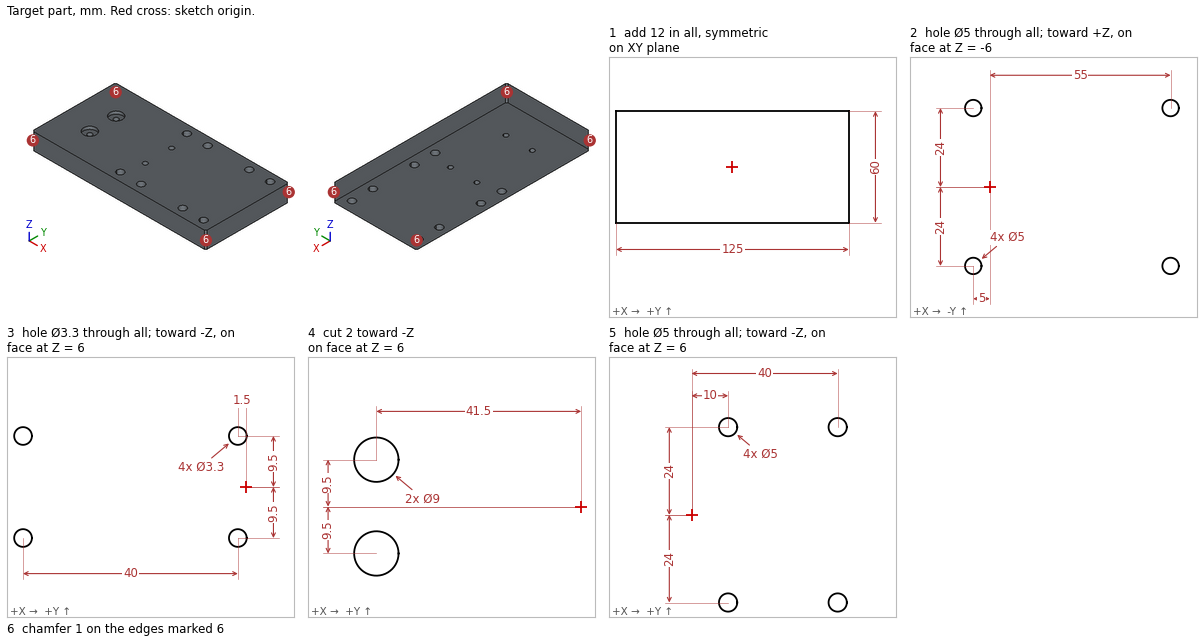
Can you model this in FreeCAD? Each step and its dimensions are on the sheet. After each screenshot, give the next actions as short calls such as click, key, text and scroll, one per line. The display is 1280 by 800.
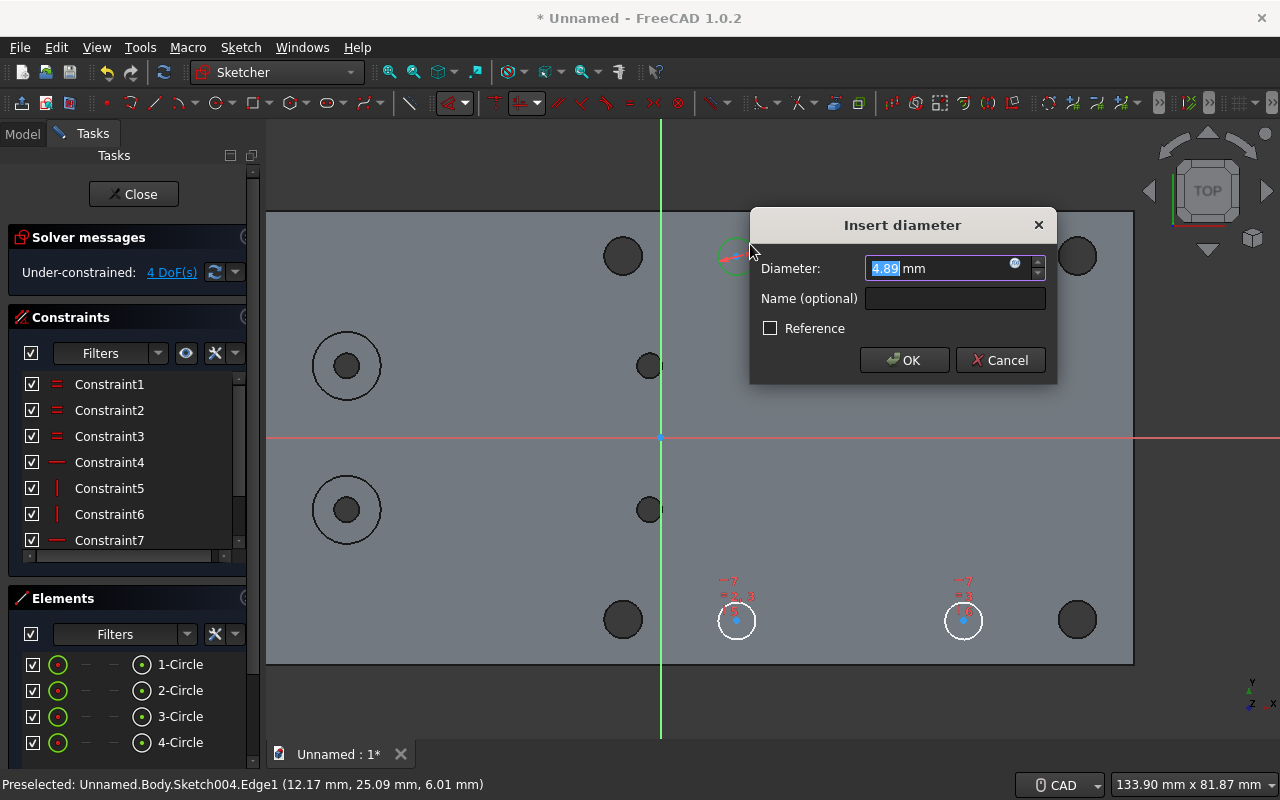
text(5)
key(Return)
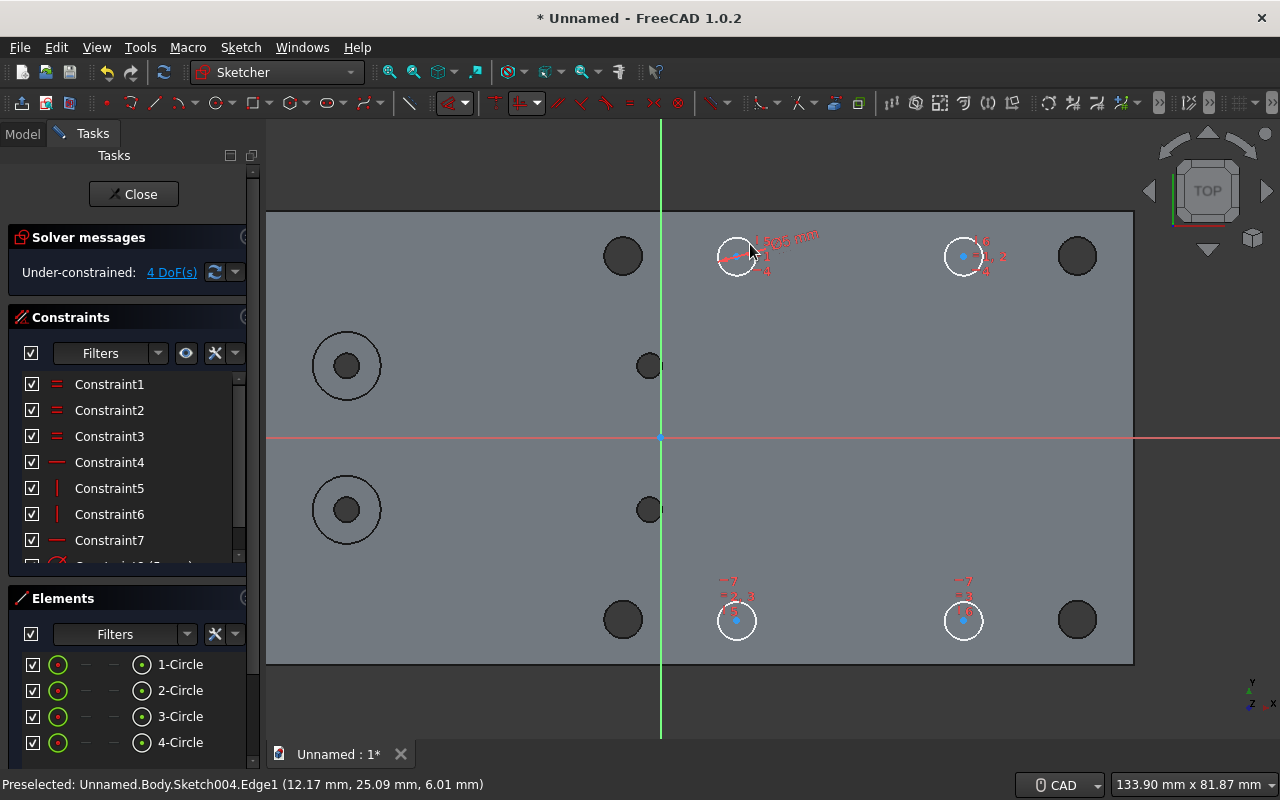
click(737, 257)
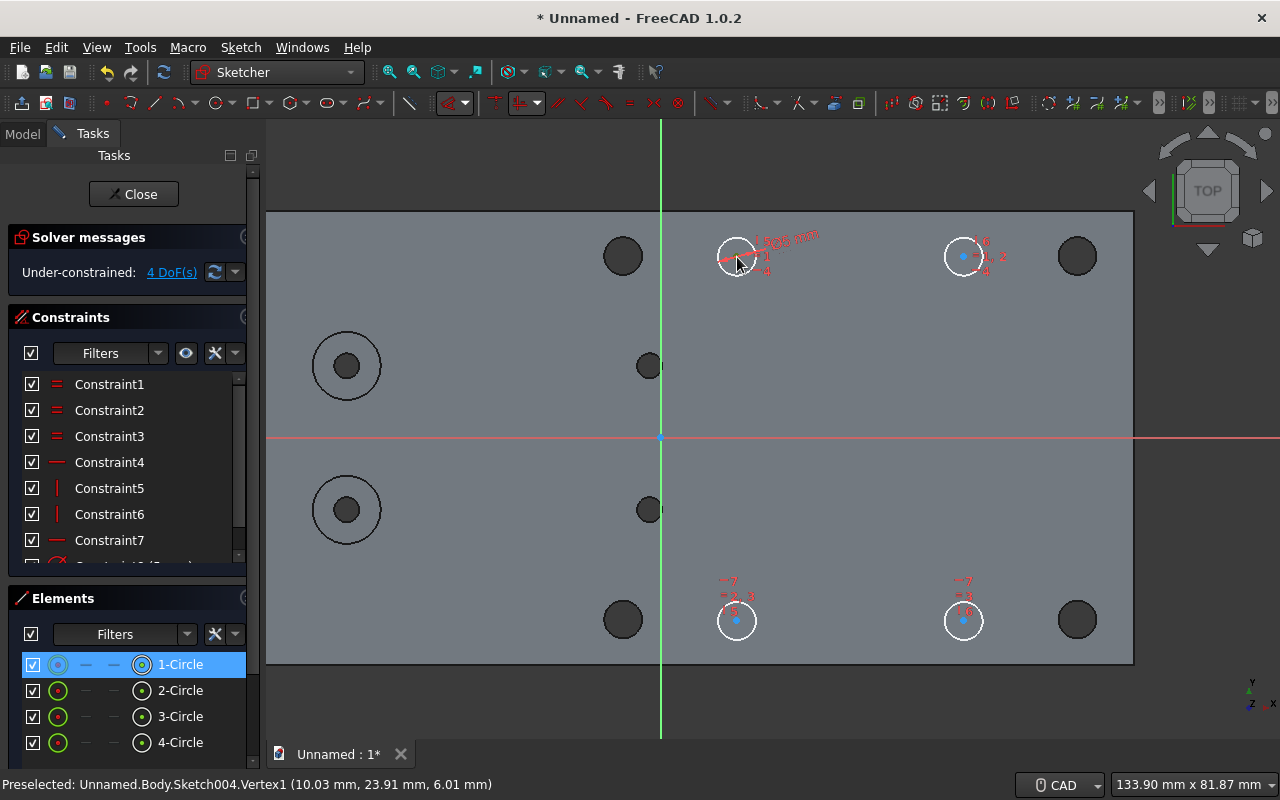
key(l)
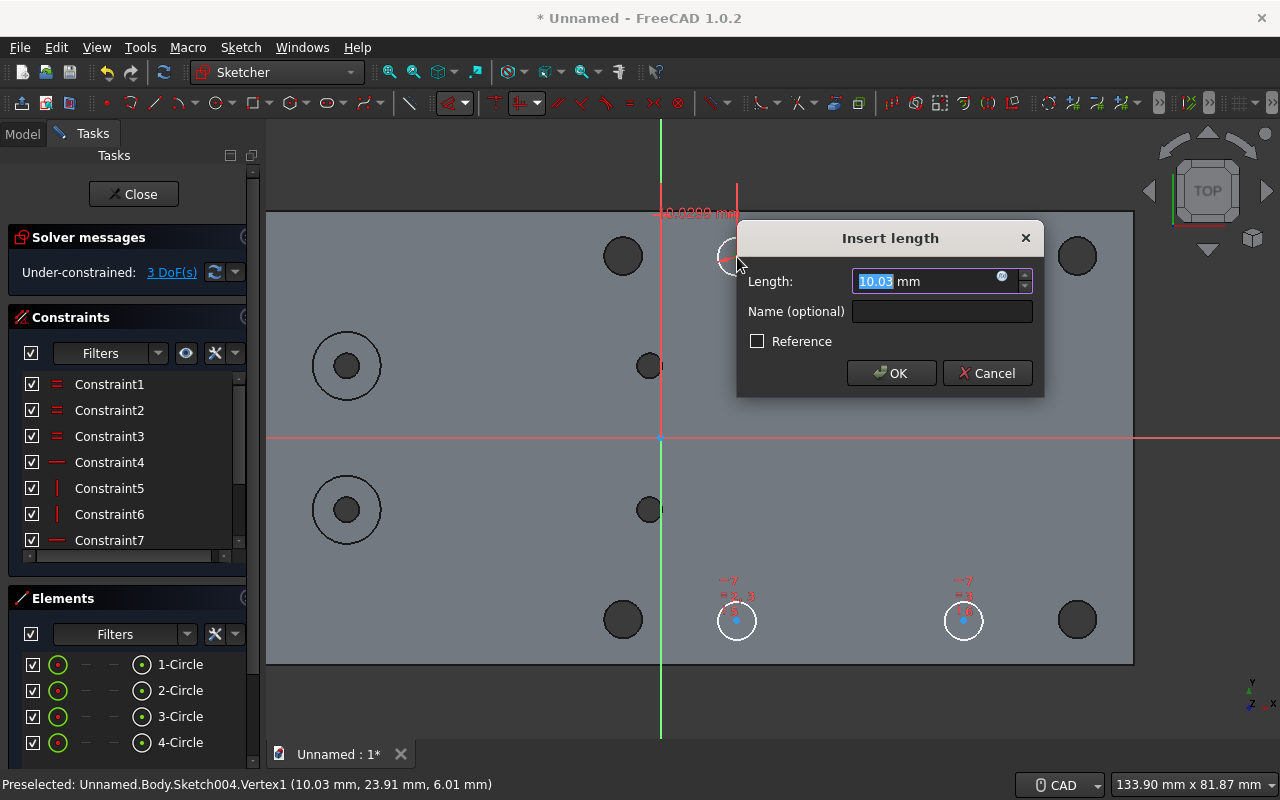
text(10)
key(Return)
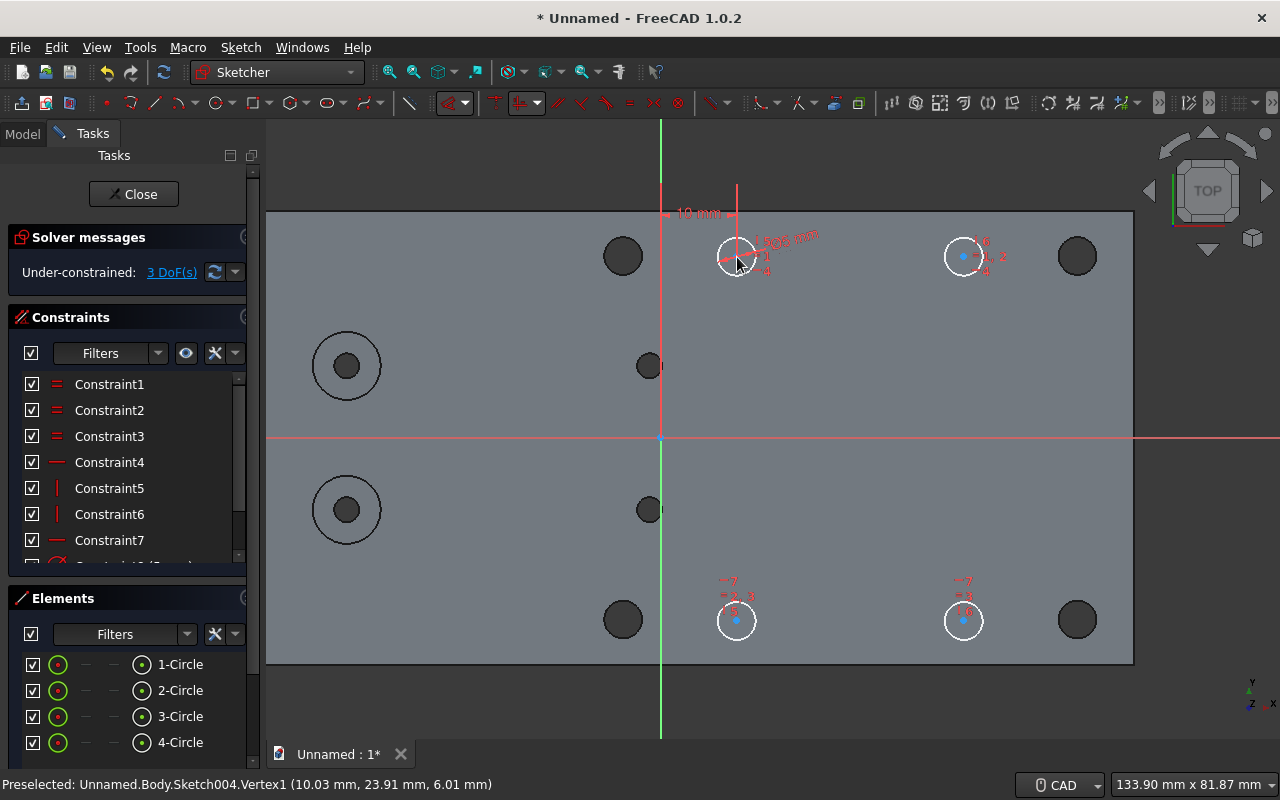
click(737, 257)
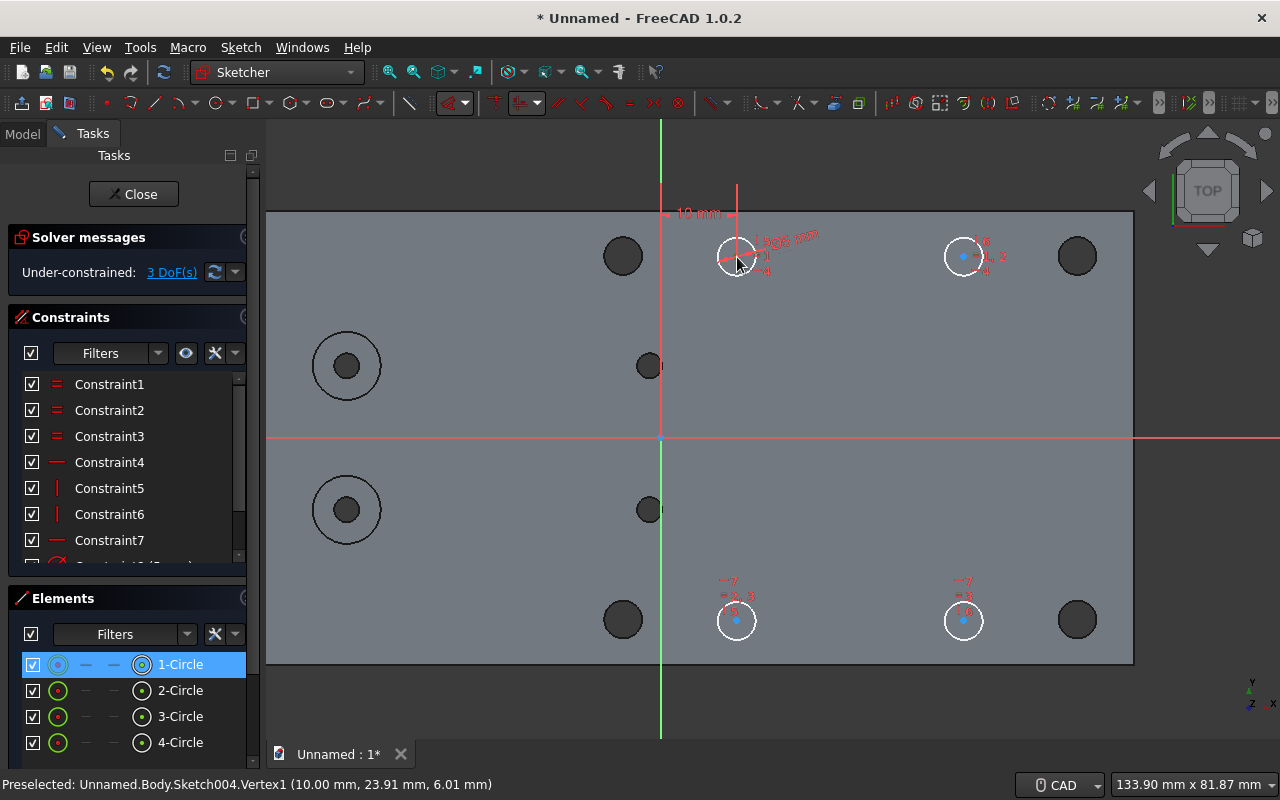
click(468, 104)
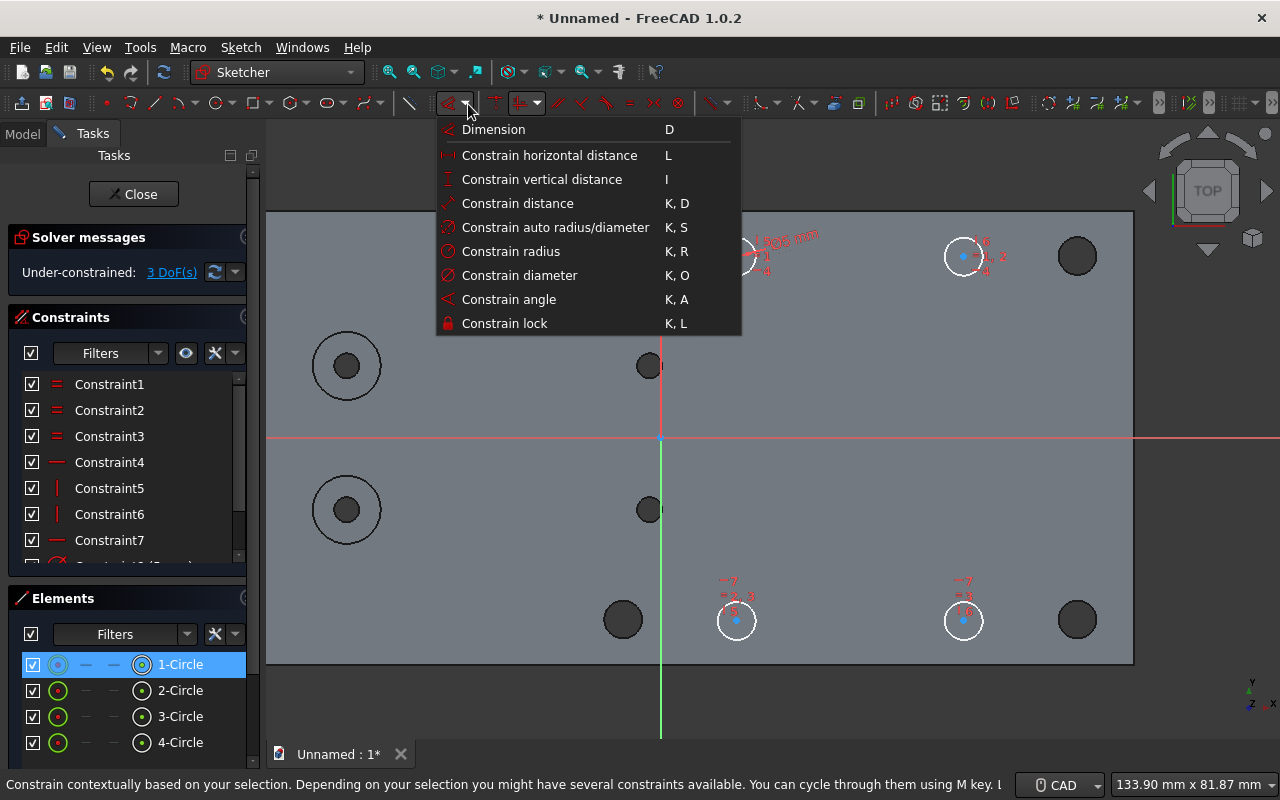
click(589, 179)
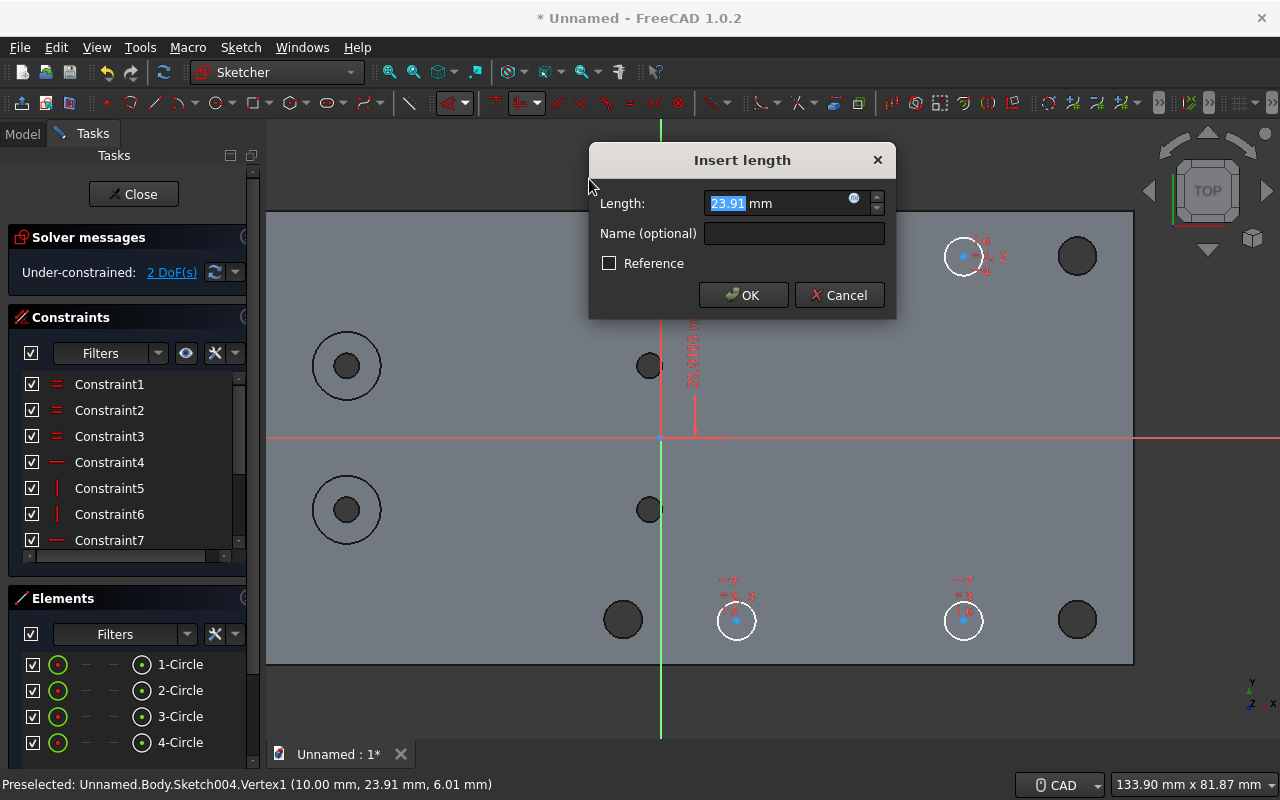
text(24)
key(Return)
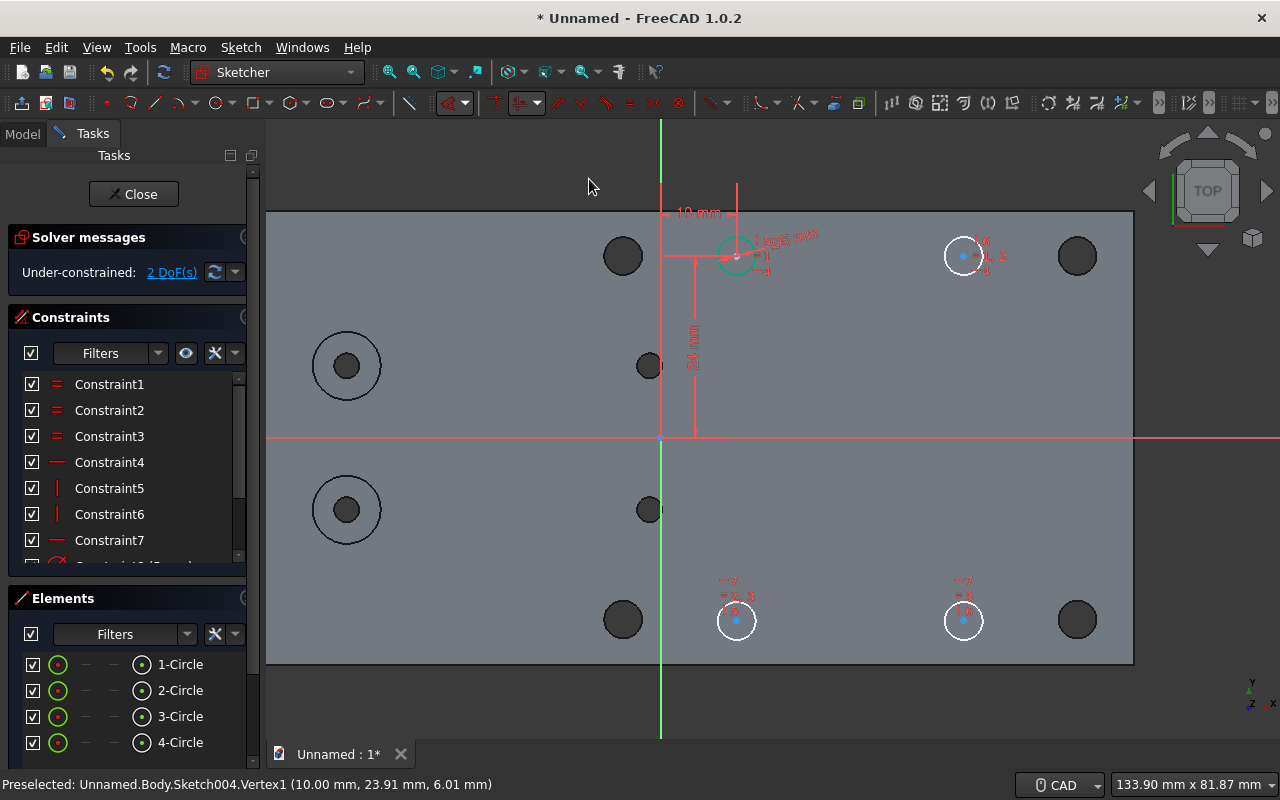
click(964, 256)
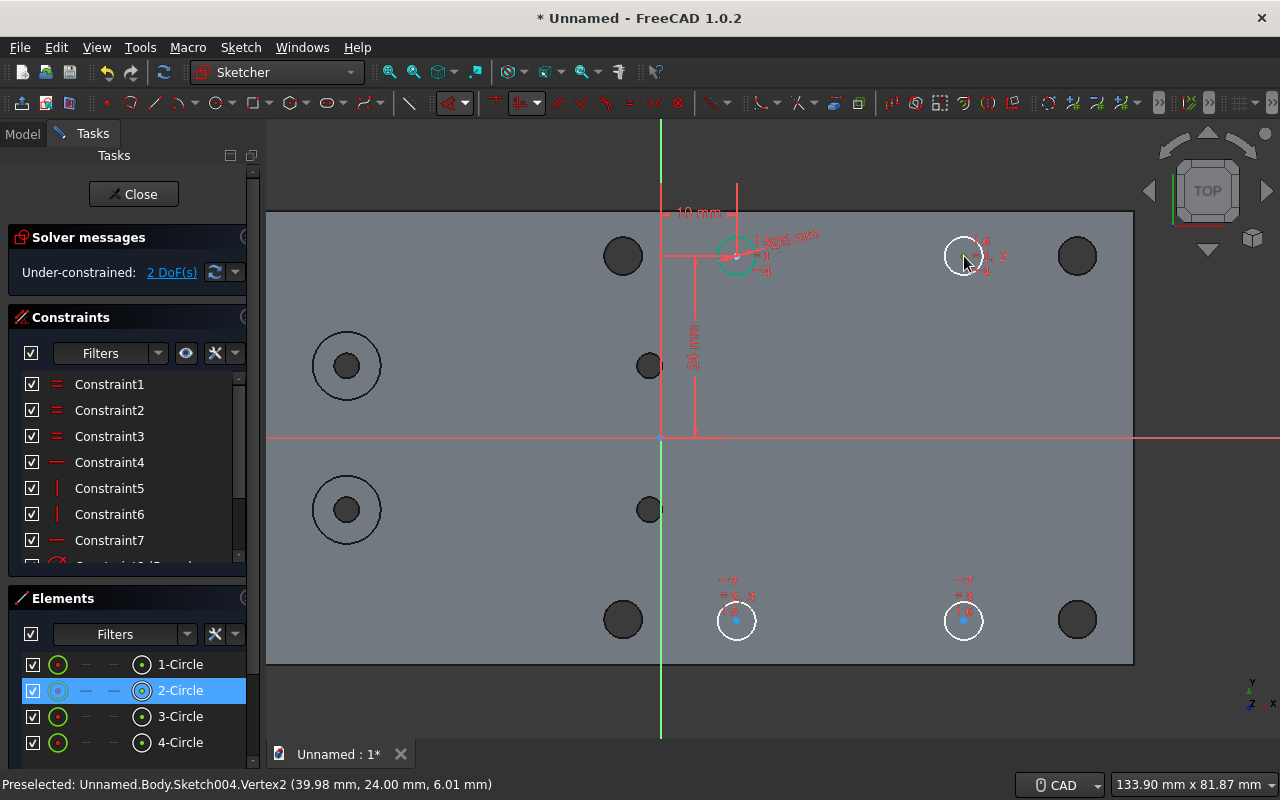
key(l)